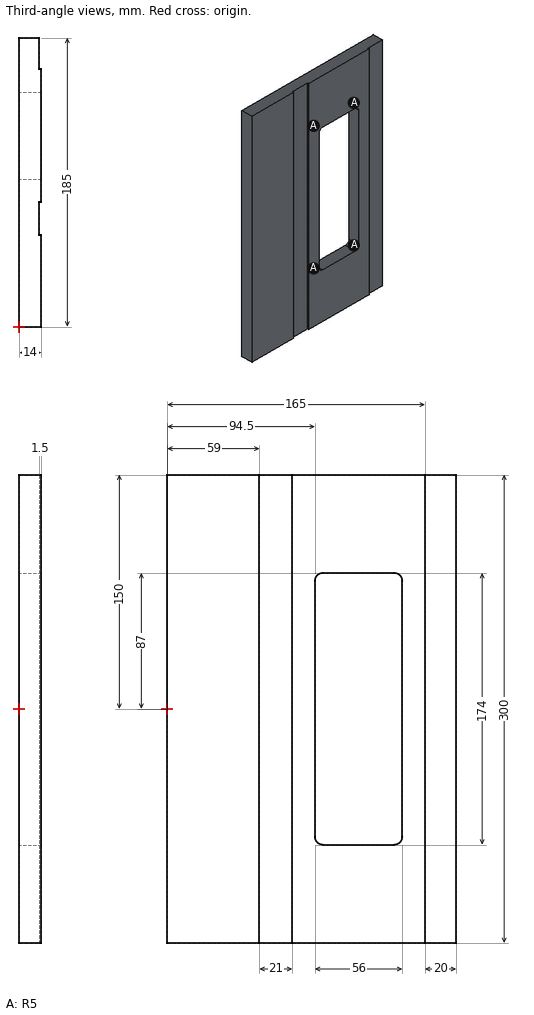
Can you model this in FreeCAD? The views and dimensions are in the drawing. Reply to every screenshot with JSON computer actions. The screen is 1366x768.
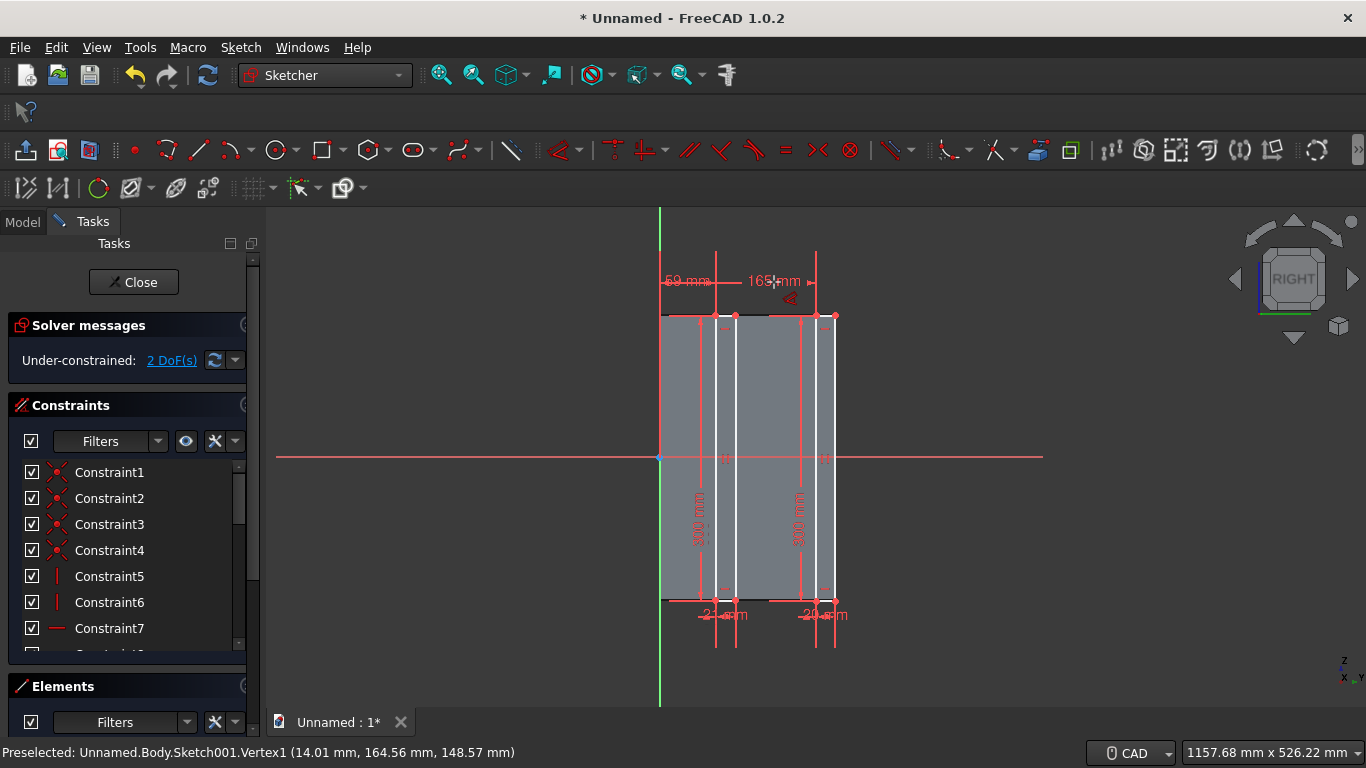
{"action": "left_click", "coordinate": [816, 316]}
{"action": "left_click", "coordinate": [626, 387]}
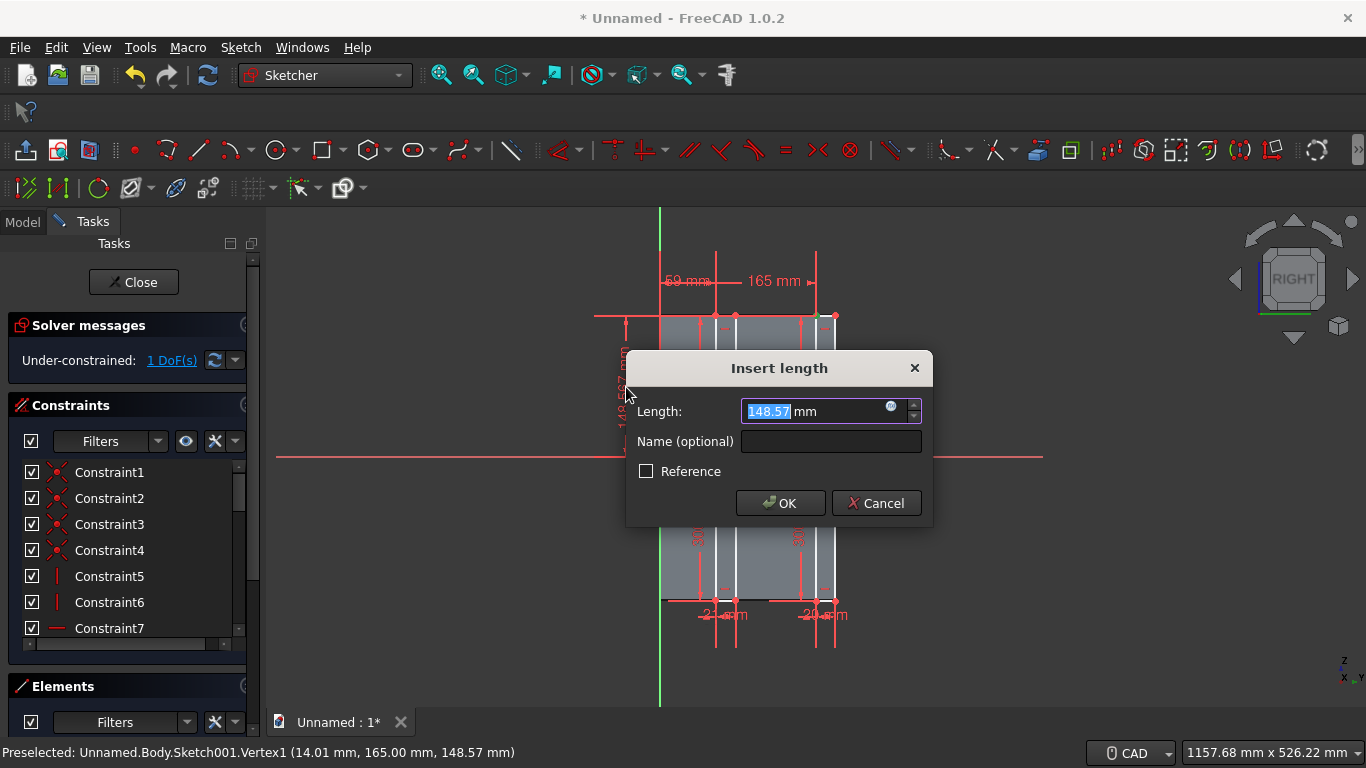
{"action": "type", "text": "150"}
{"action": "key", "text": "Return"}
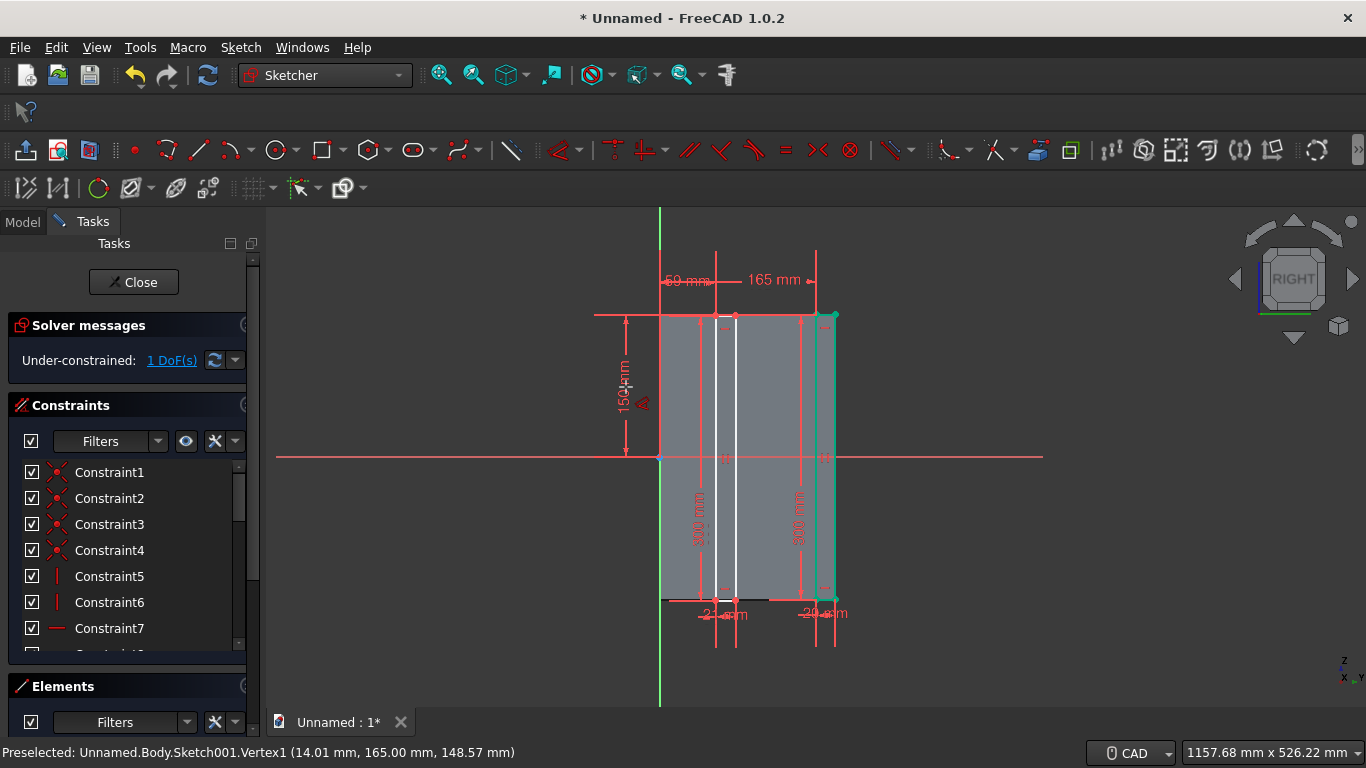
{"action": "left_click", "coordinate": [716, 316]}
{"action": "left_click", "coordinate": [626, 354]}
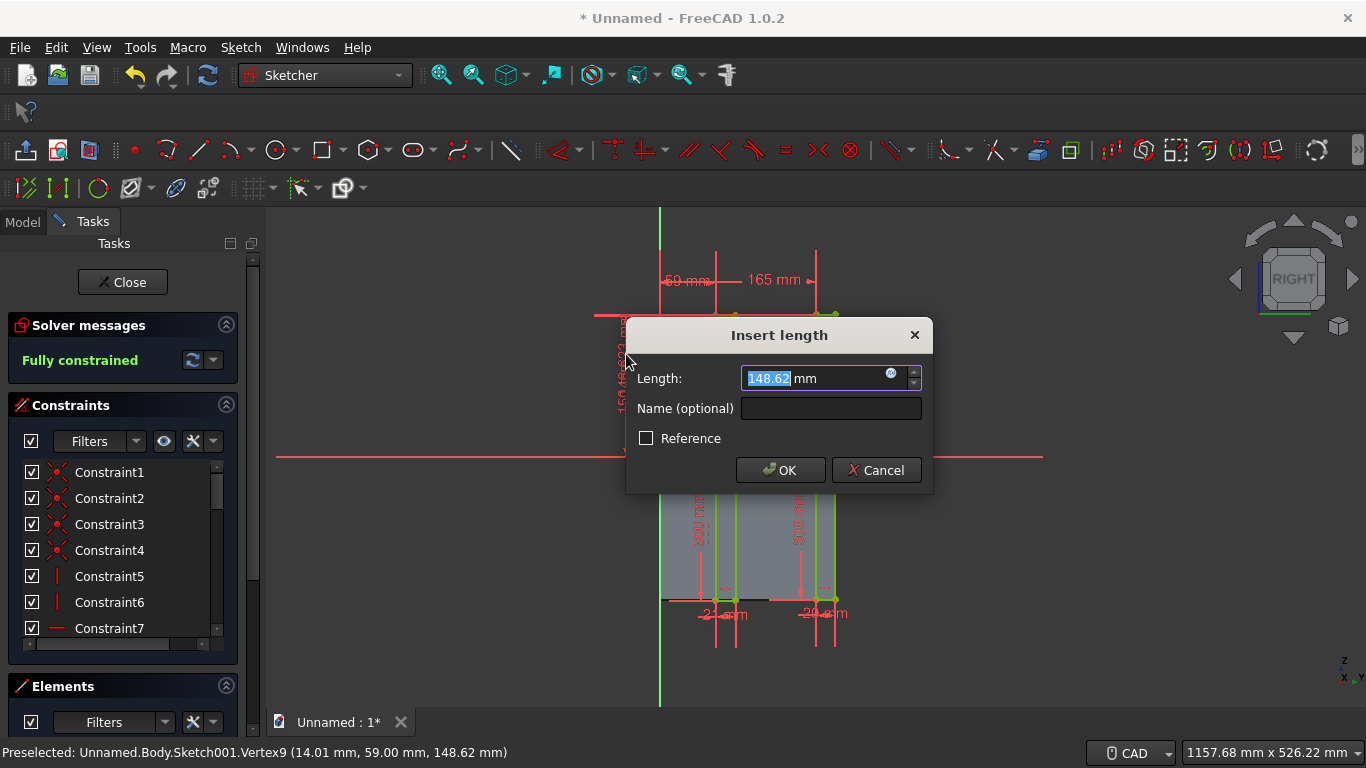
{"action": "type", "text": "150"}
{"action": "key", "text": "Return"}
{"action": "key", "text": "Escape"}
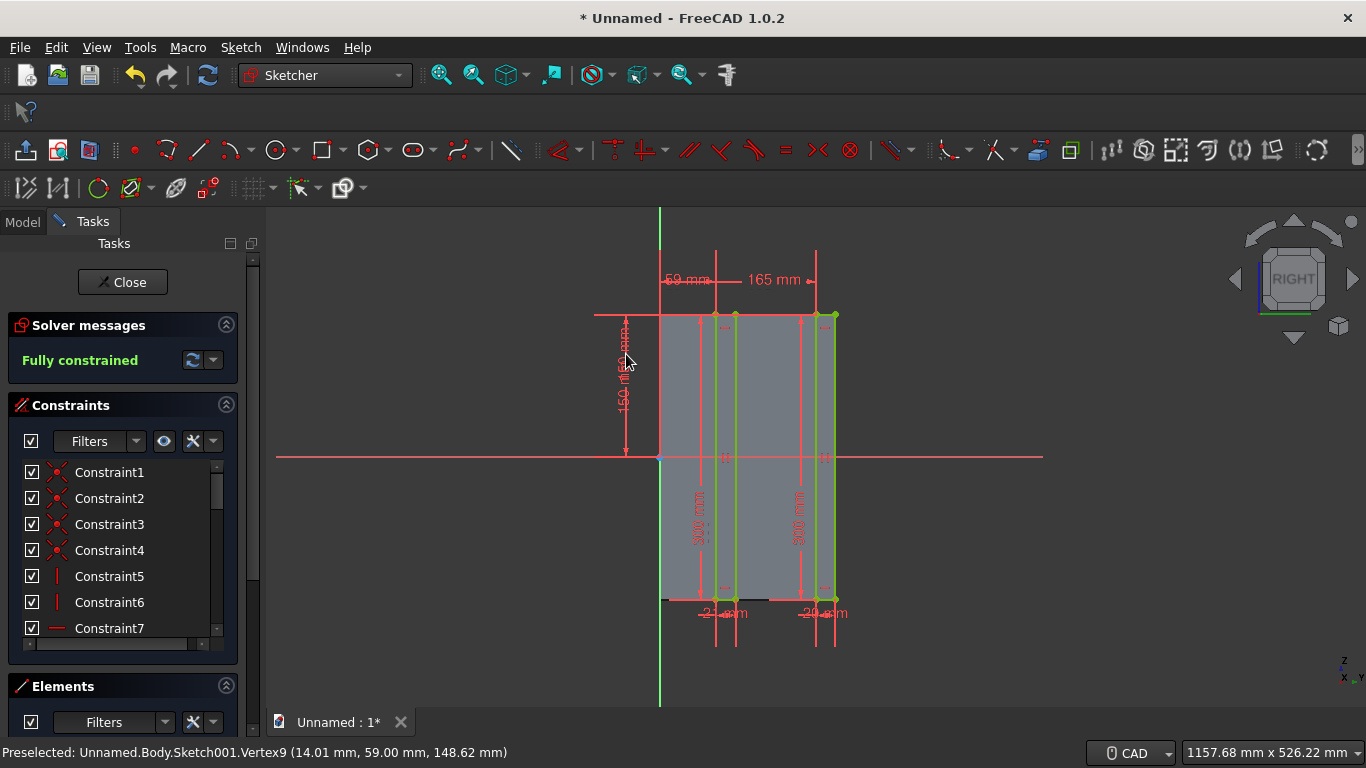
{"action": "left_click", "coordinate": [123, 282]}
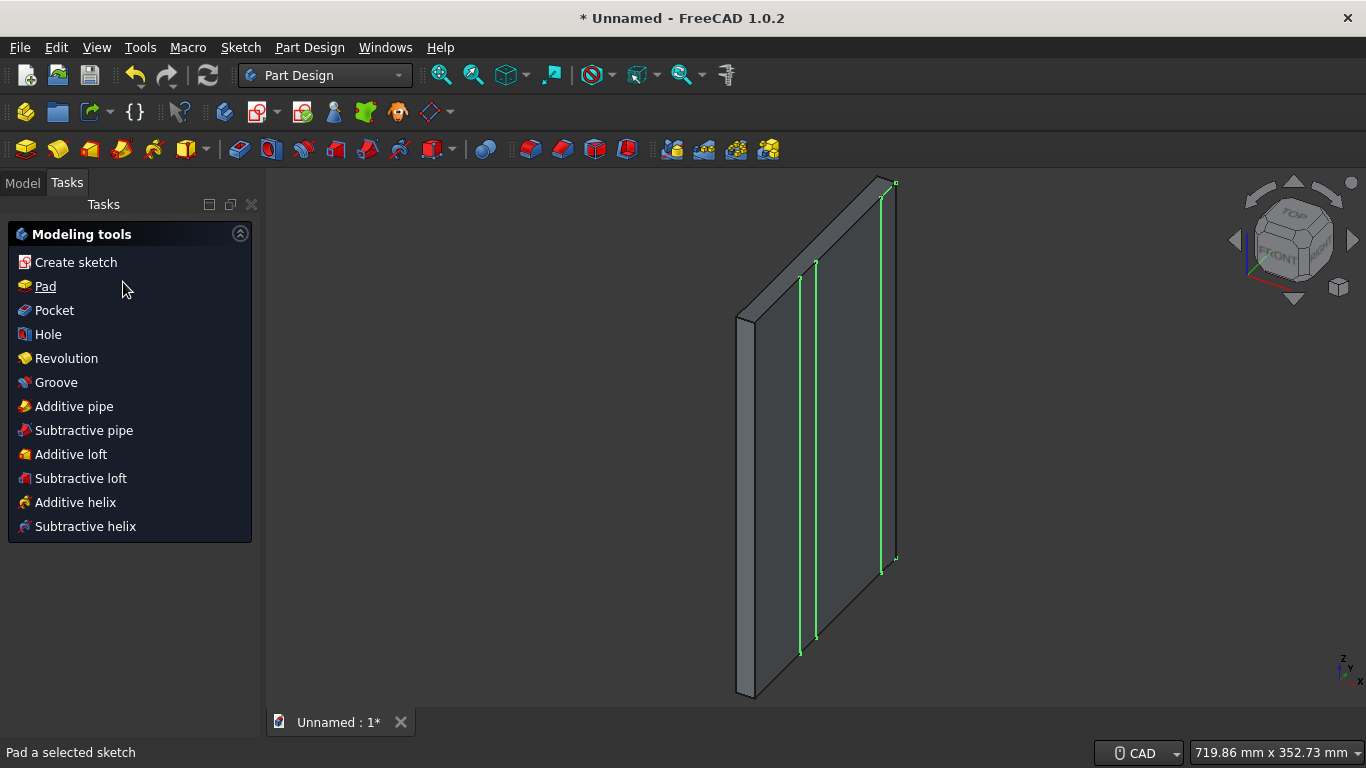
{"action": "left_click", "coordinate": [240, 150]}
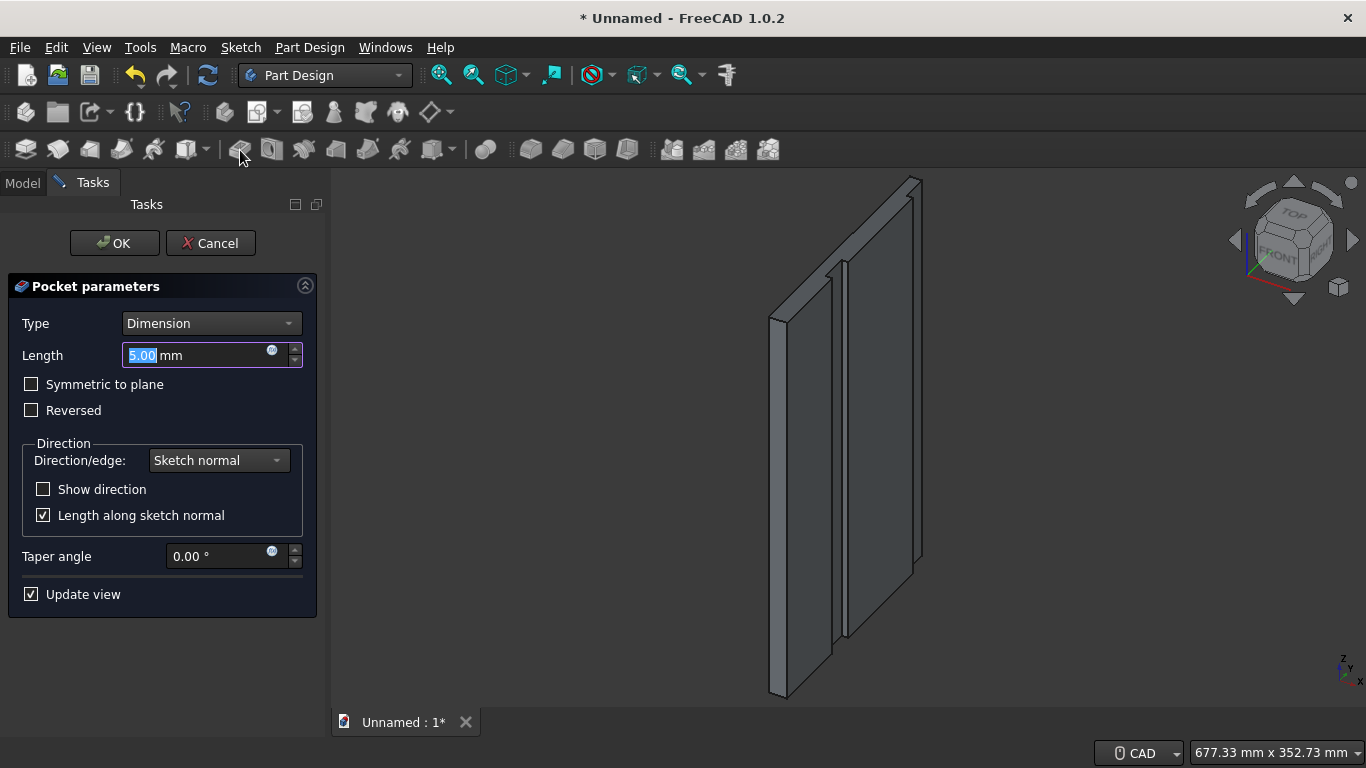
{"action": "type", "text": "1.5"}
{"action": "key", "text": "Tab"}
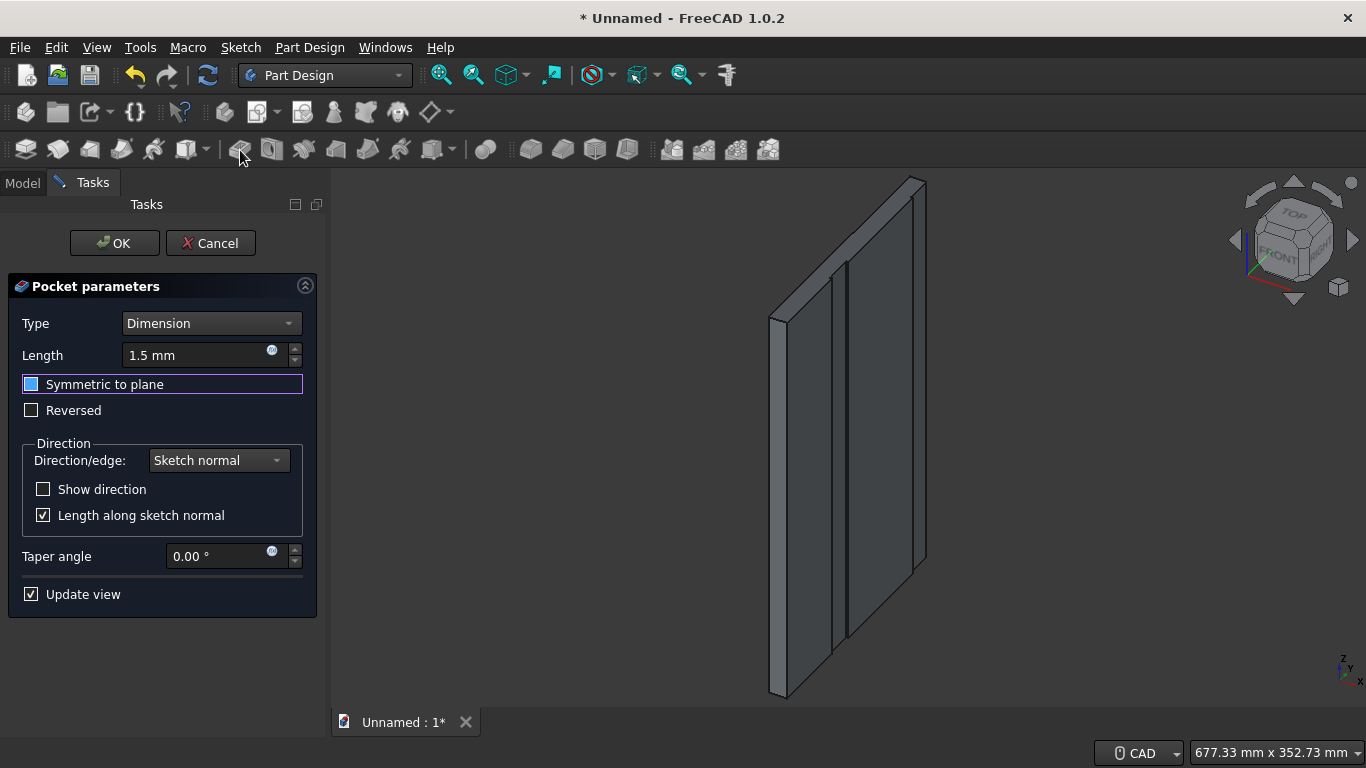
{"action": "left_click", "coordinate": [115, 243]}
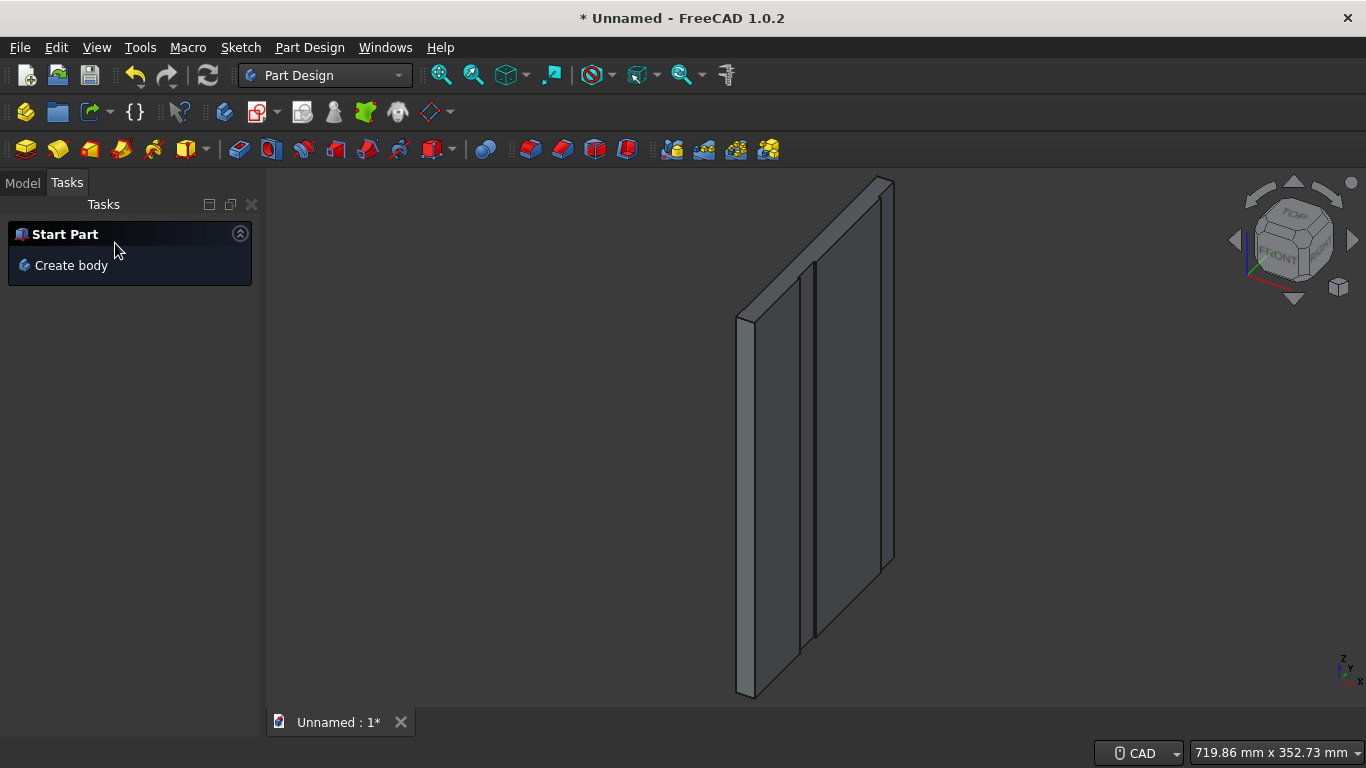
{"action": "left_click", "coordinate": [848, 310]}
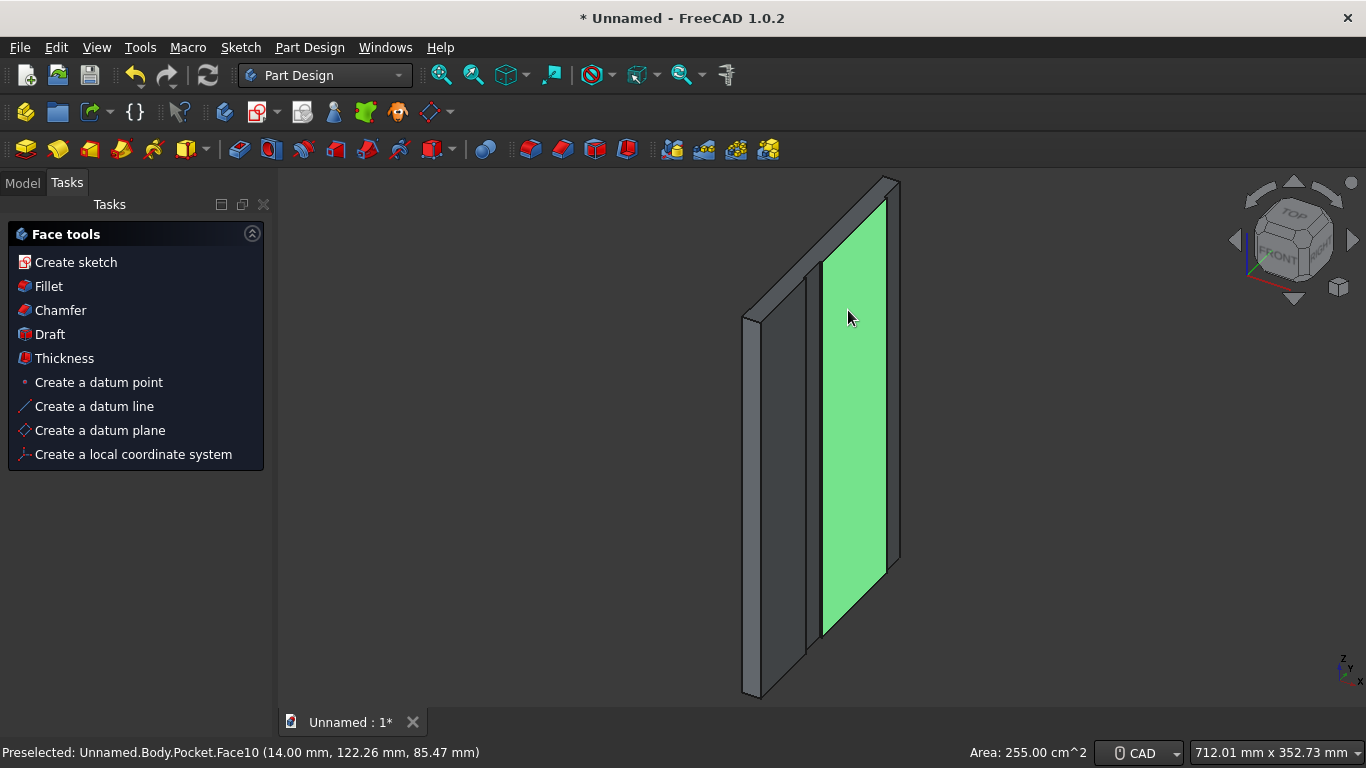
{"action": "left_click", "coordinate": [258, 112]}